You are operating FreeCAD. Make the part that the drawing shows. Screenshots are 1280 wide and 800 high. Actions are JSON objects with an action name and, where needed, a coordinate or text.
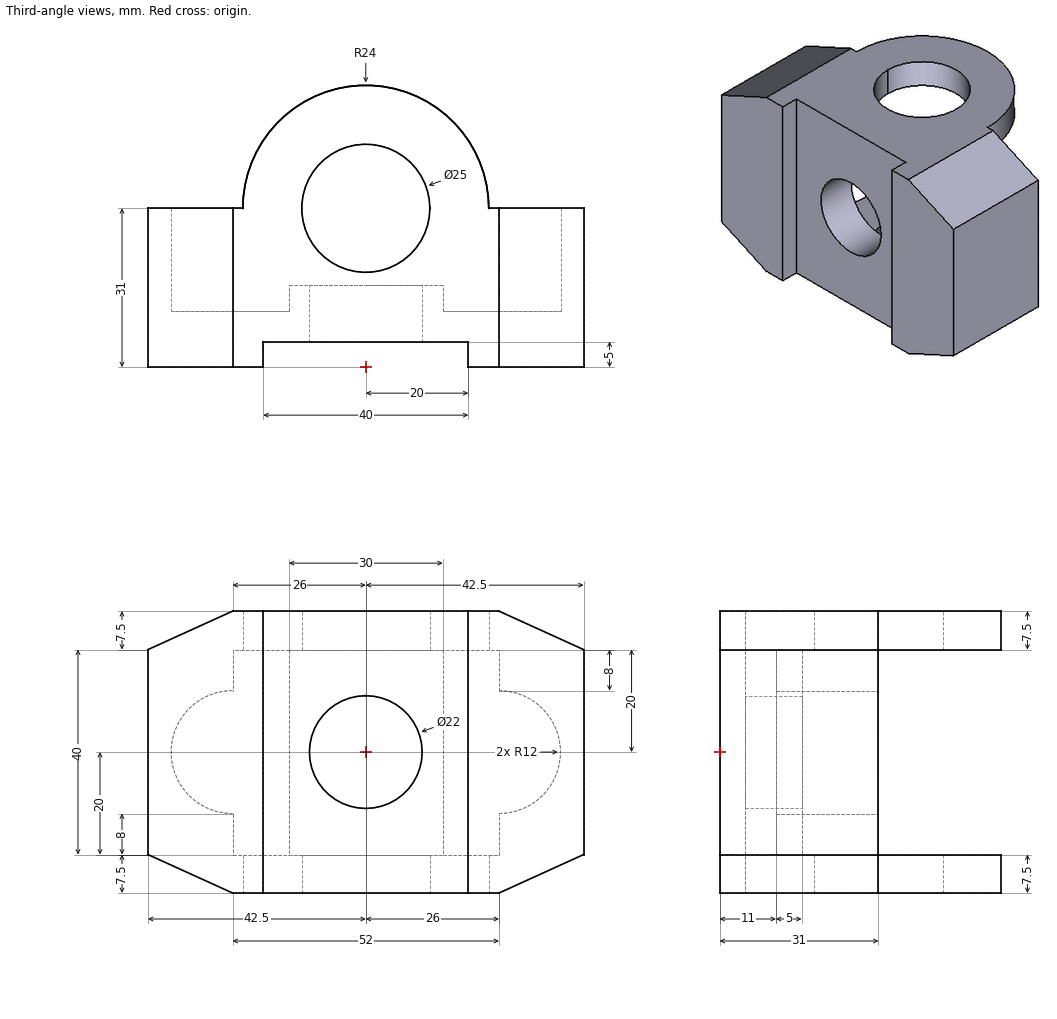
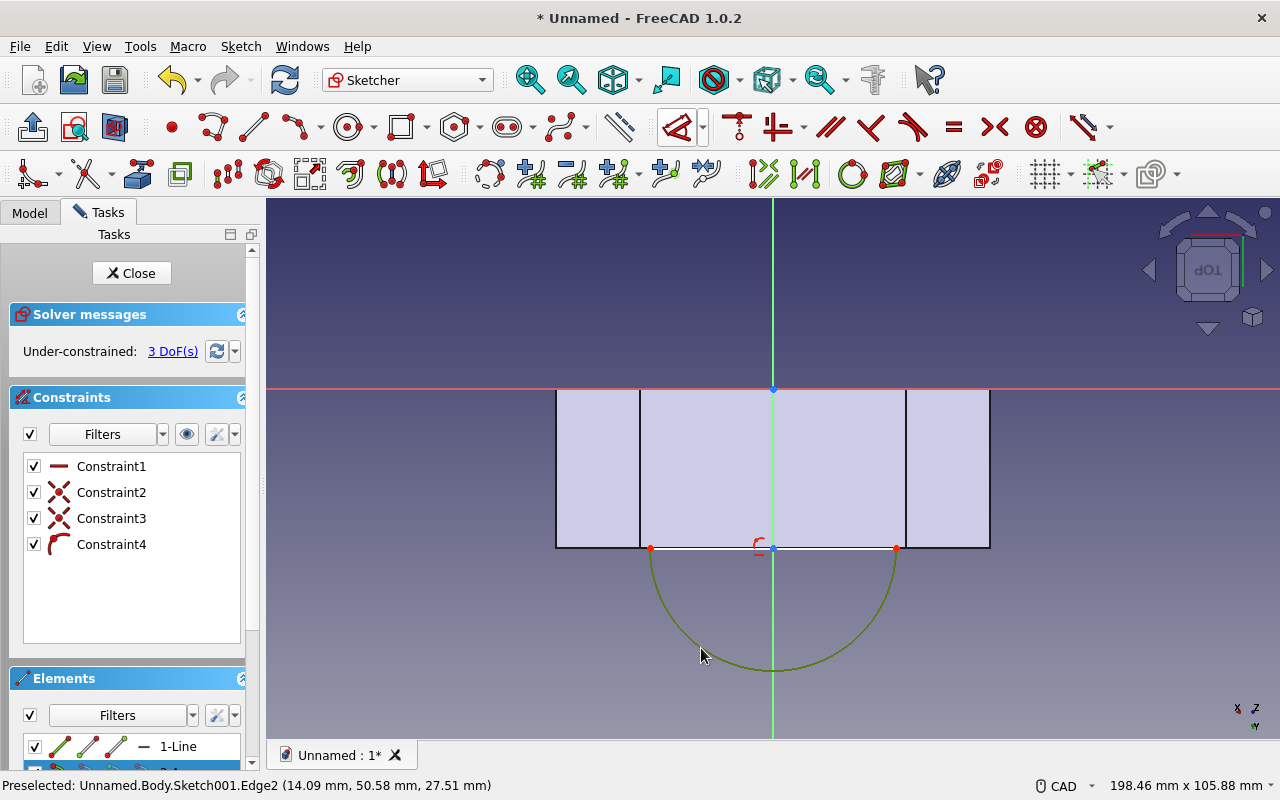
{"action": "key", "text": "k r"}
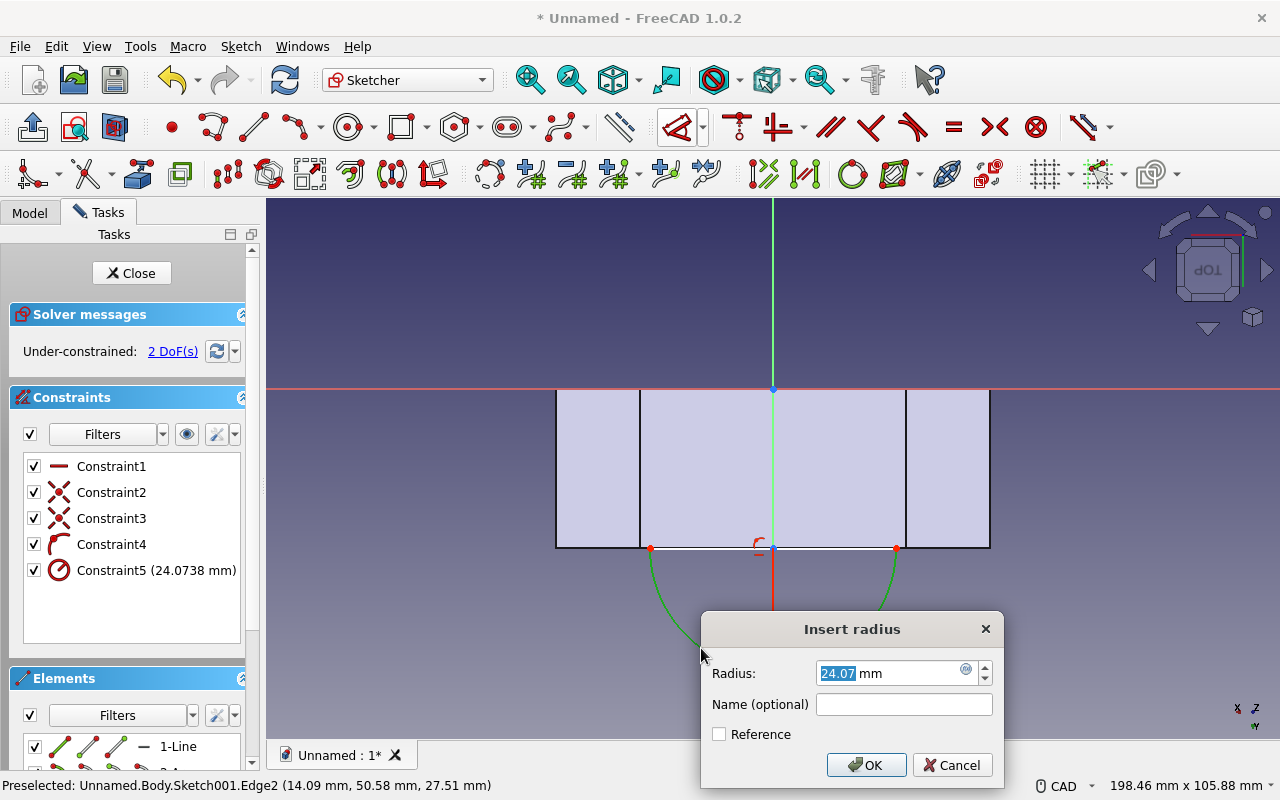
{"action": "type", "text": "24"}
{"action": "key", "text": "Return"}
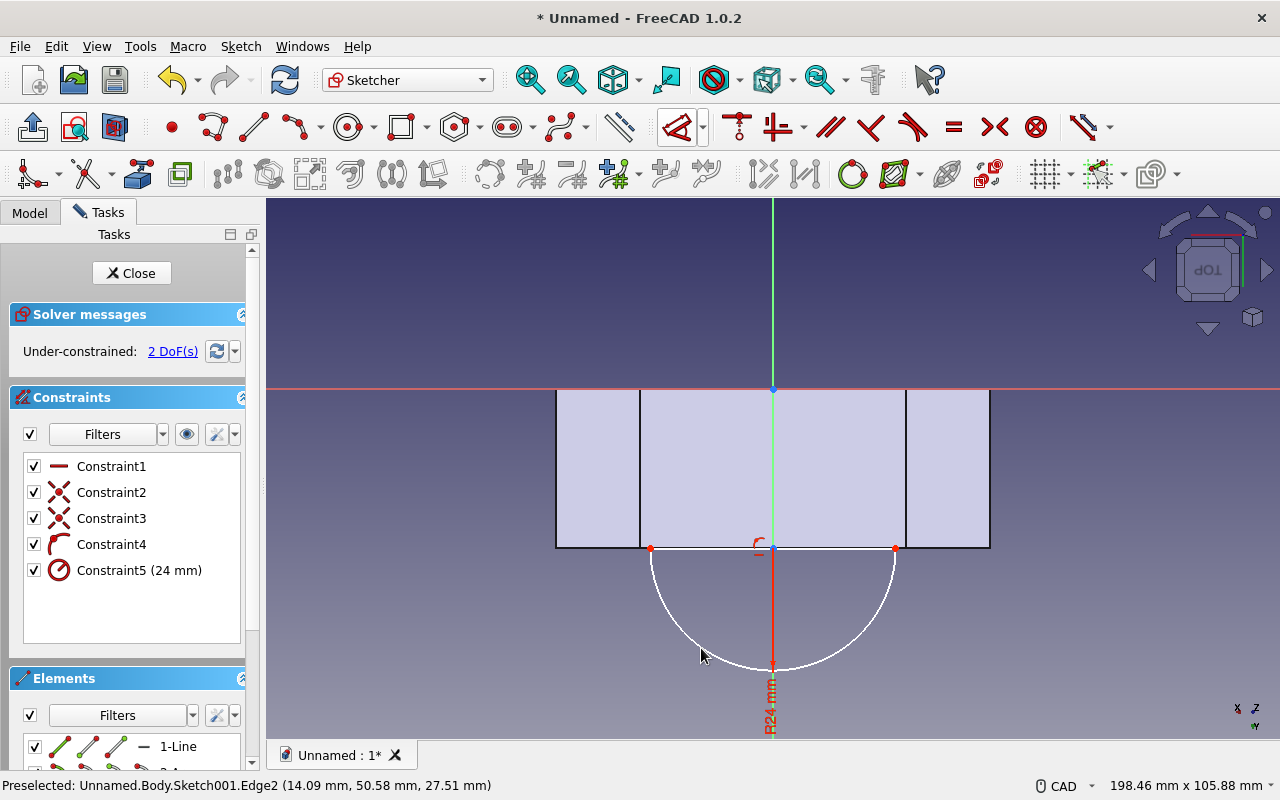
{"action": "left_click", "coordinate": [896, 549]}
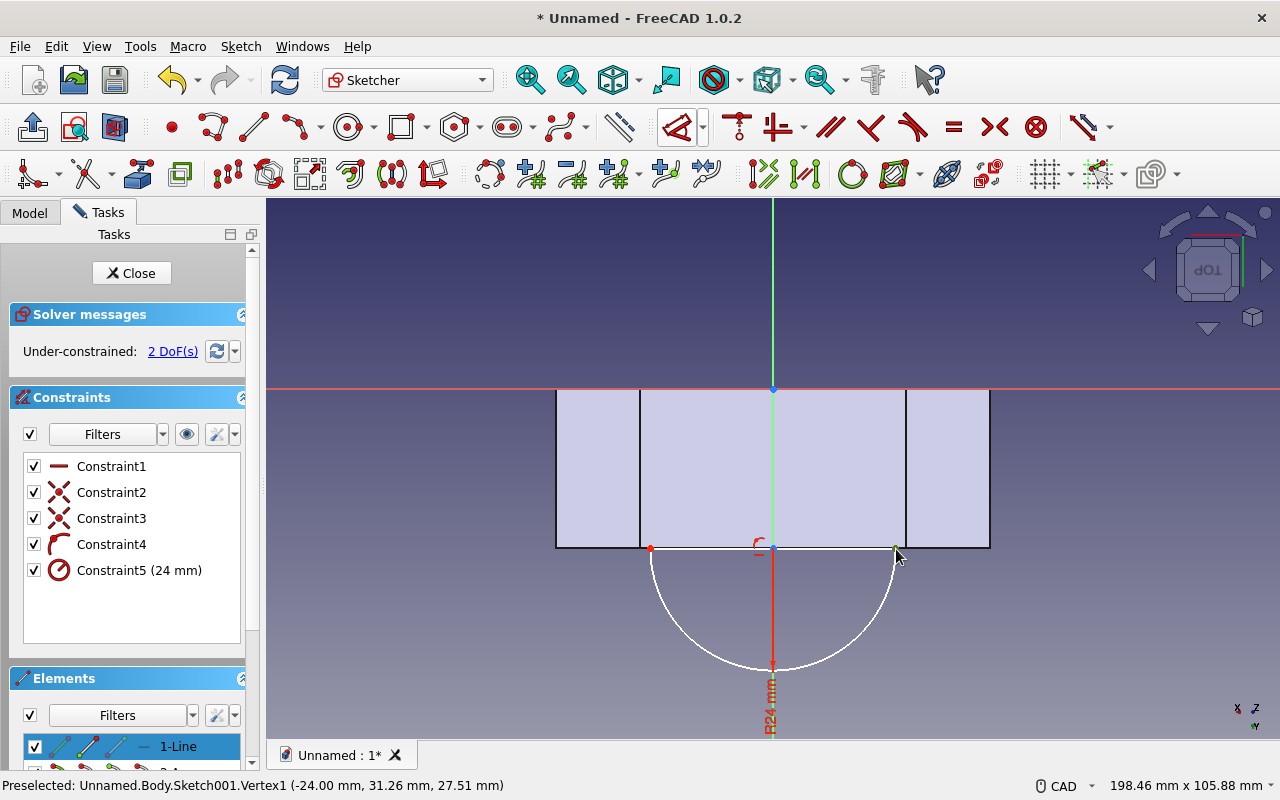
{"action": "key", "text": "i"}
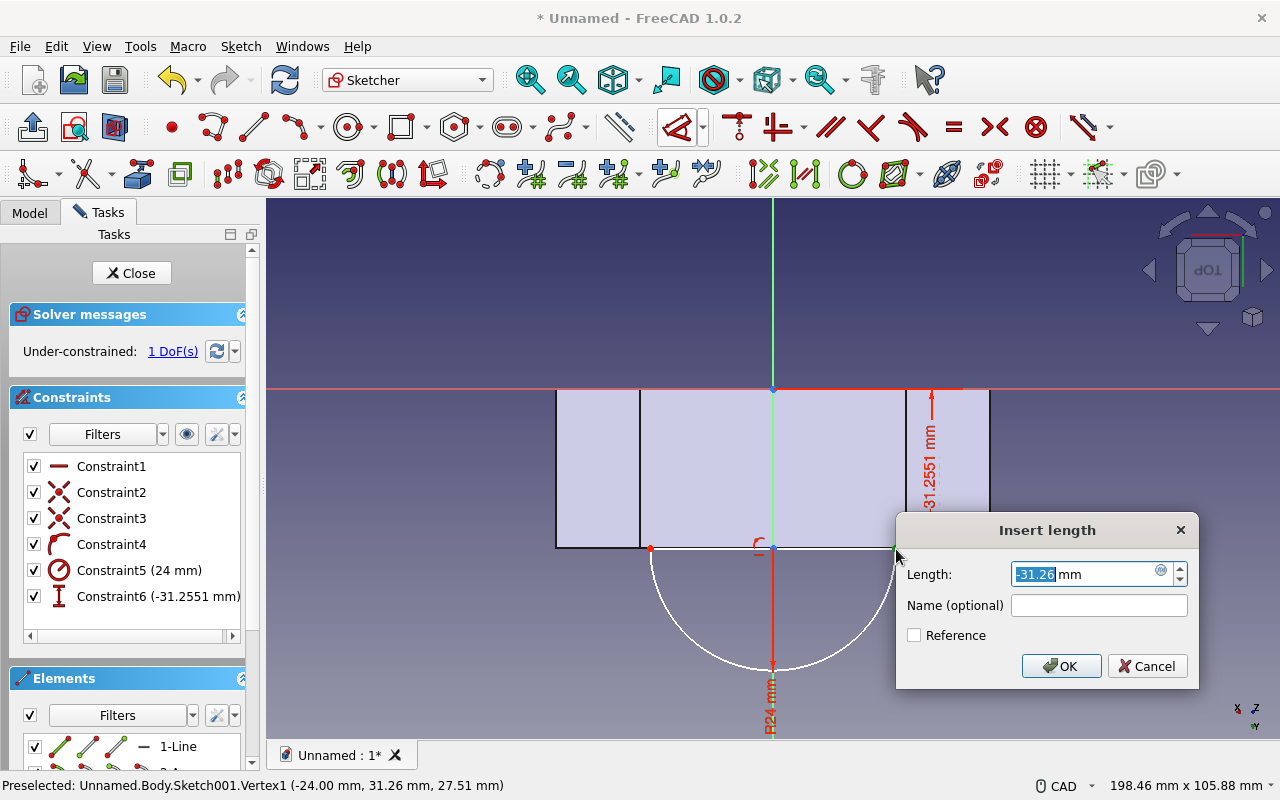
{"action": "type", "text": "-31"}
{"action": "key", "text": "Return"}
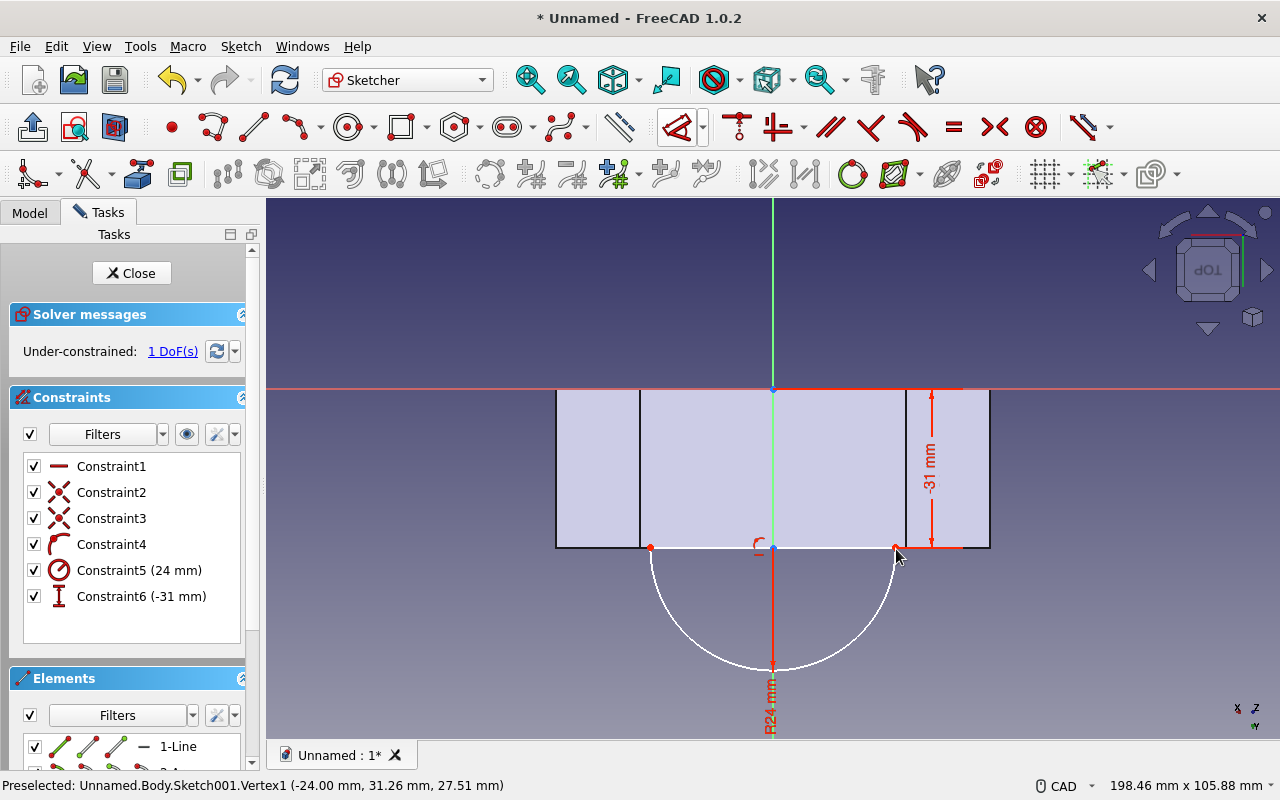
{"action": "left_click", "coordinate": [773, 548]}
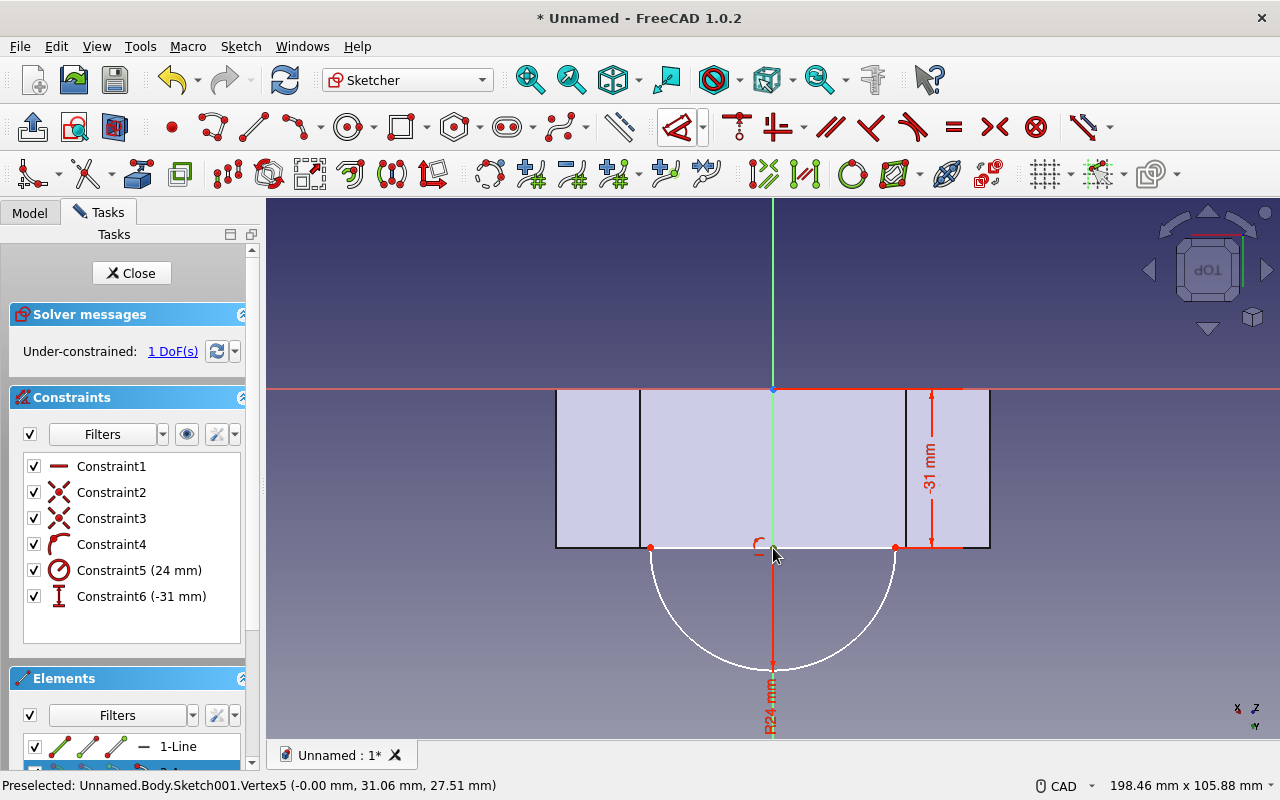
{"action": "key", "text": "i"}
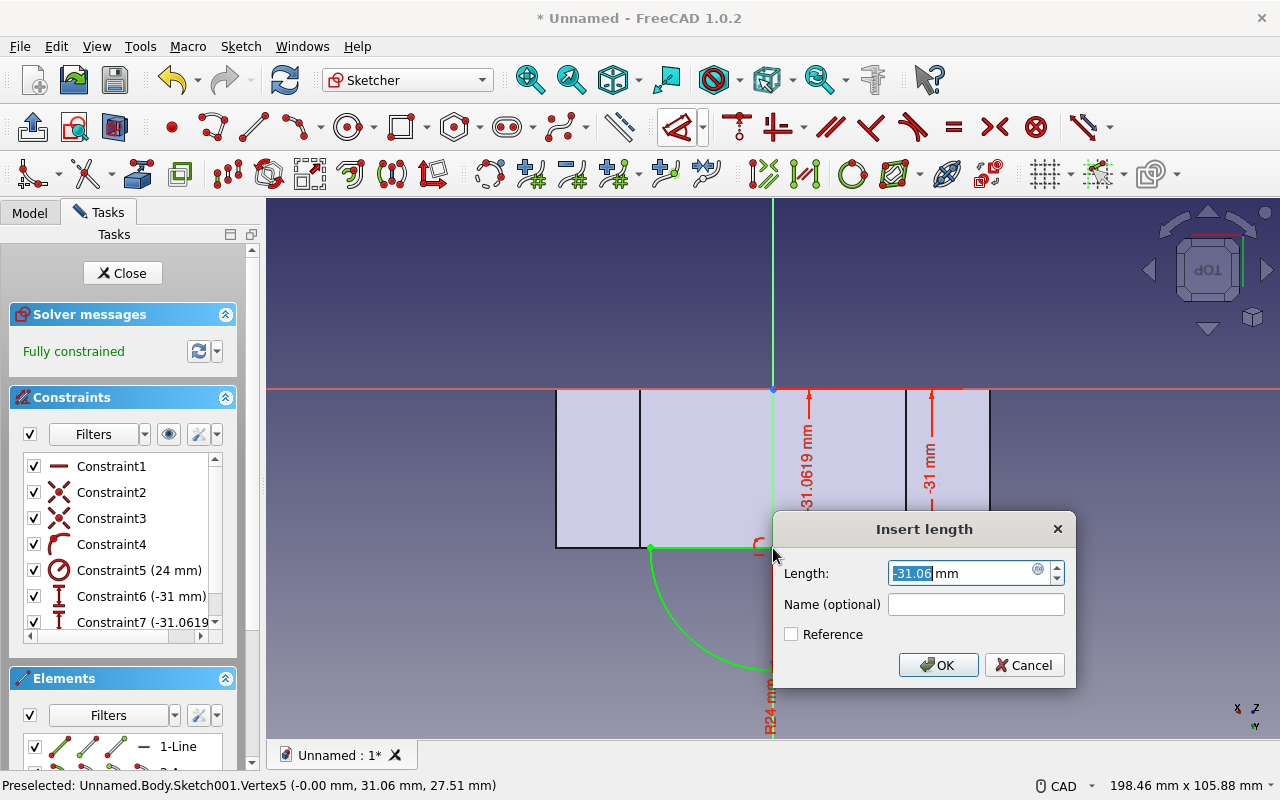
{"action": "type", "text": "-31"}
{"action": "key", "text": "Return"}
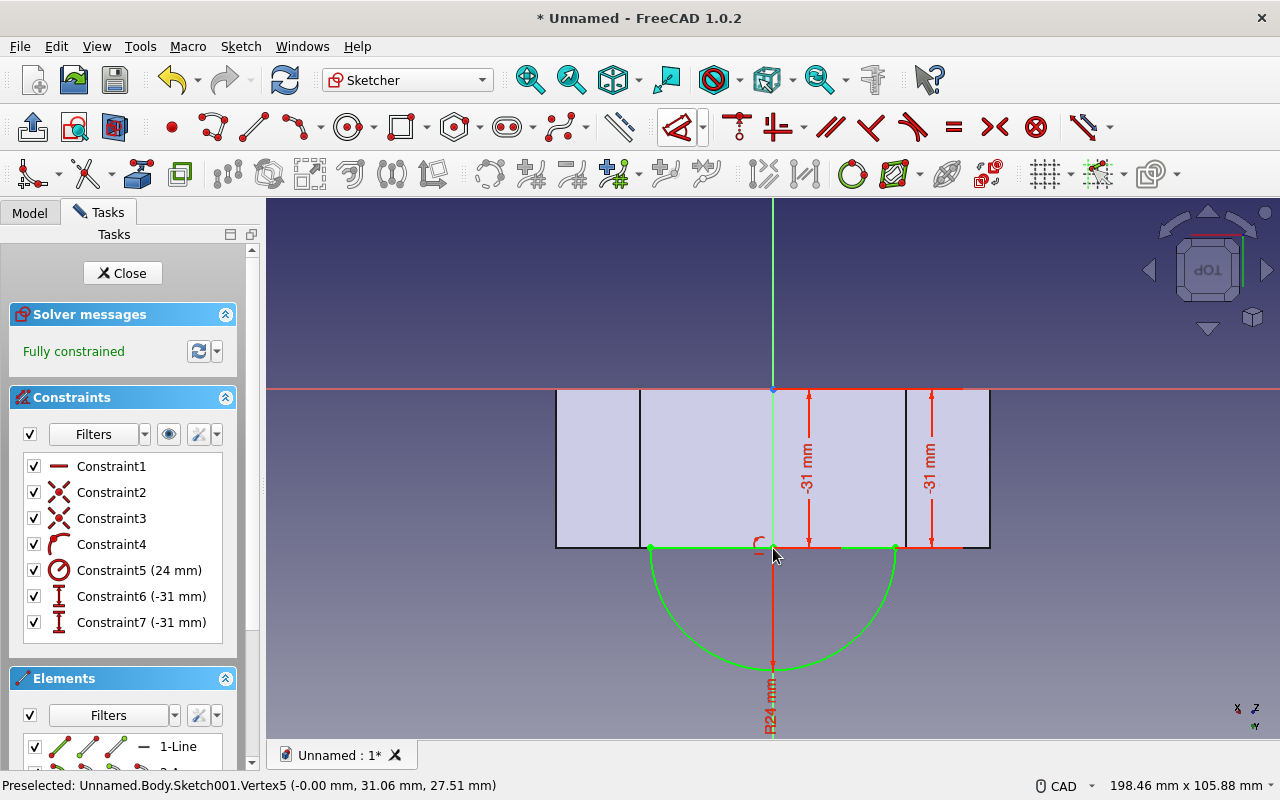
{"action": "left_click", "coordinate": [123, 273]}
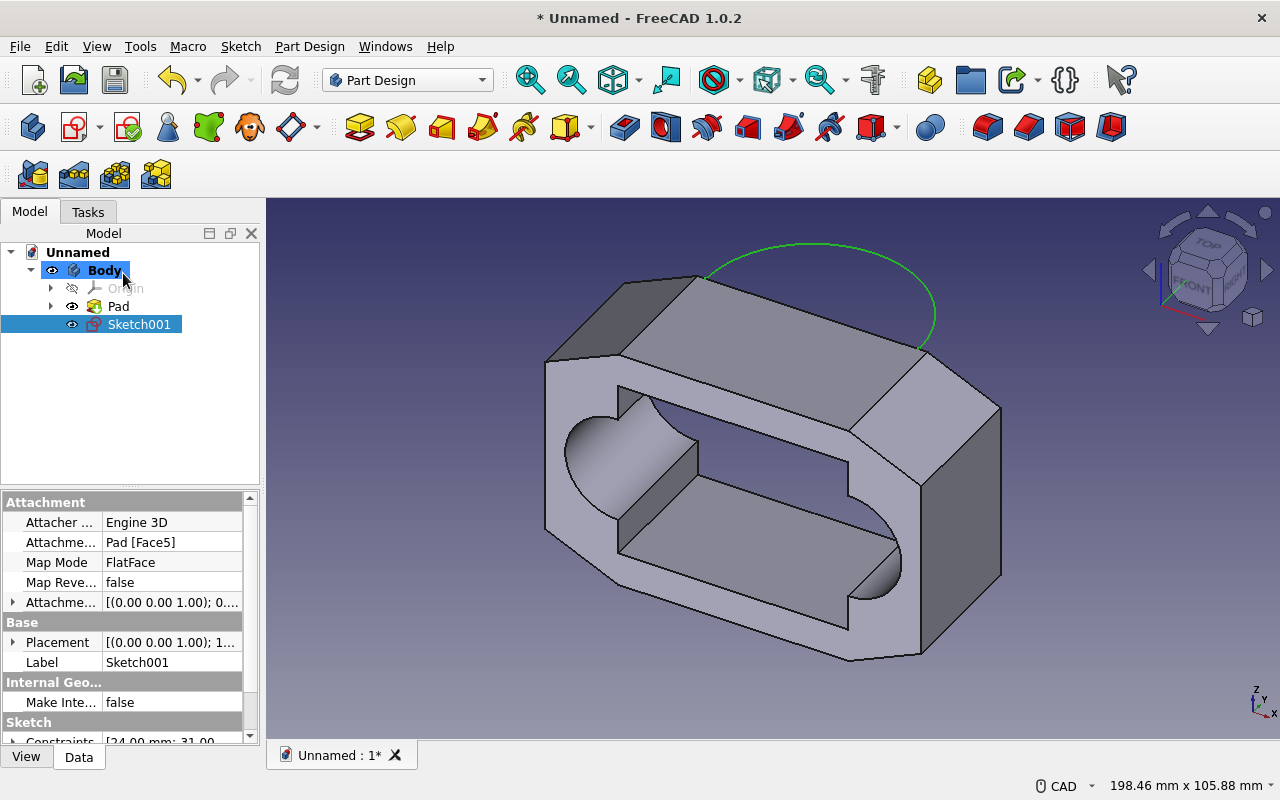
{"action": "left_click", "coordinate": [360, 128]}